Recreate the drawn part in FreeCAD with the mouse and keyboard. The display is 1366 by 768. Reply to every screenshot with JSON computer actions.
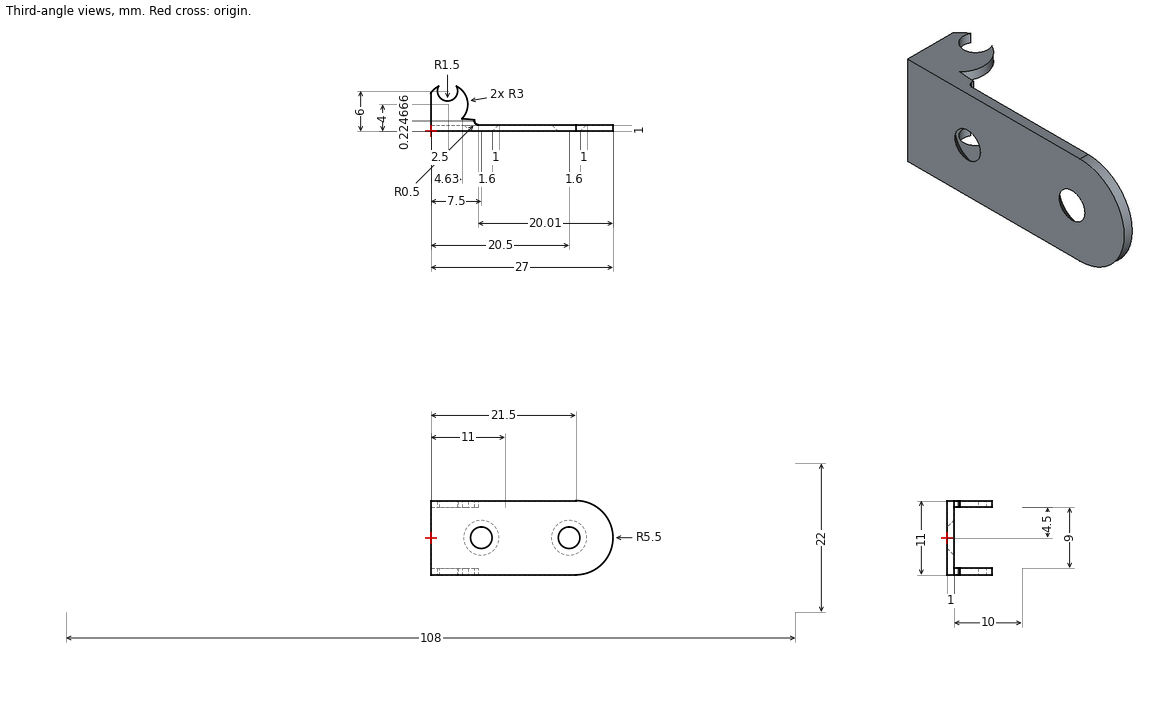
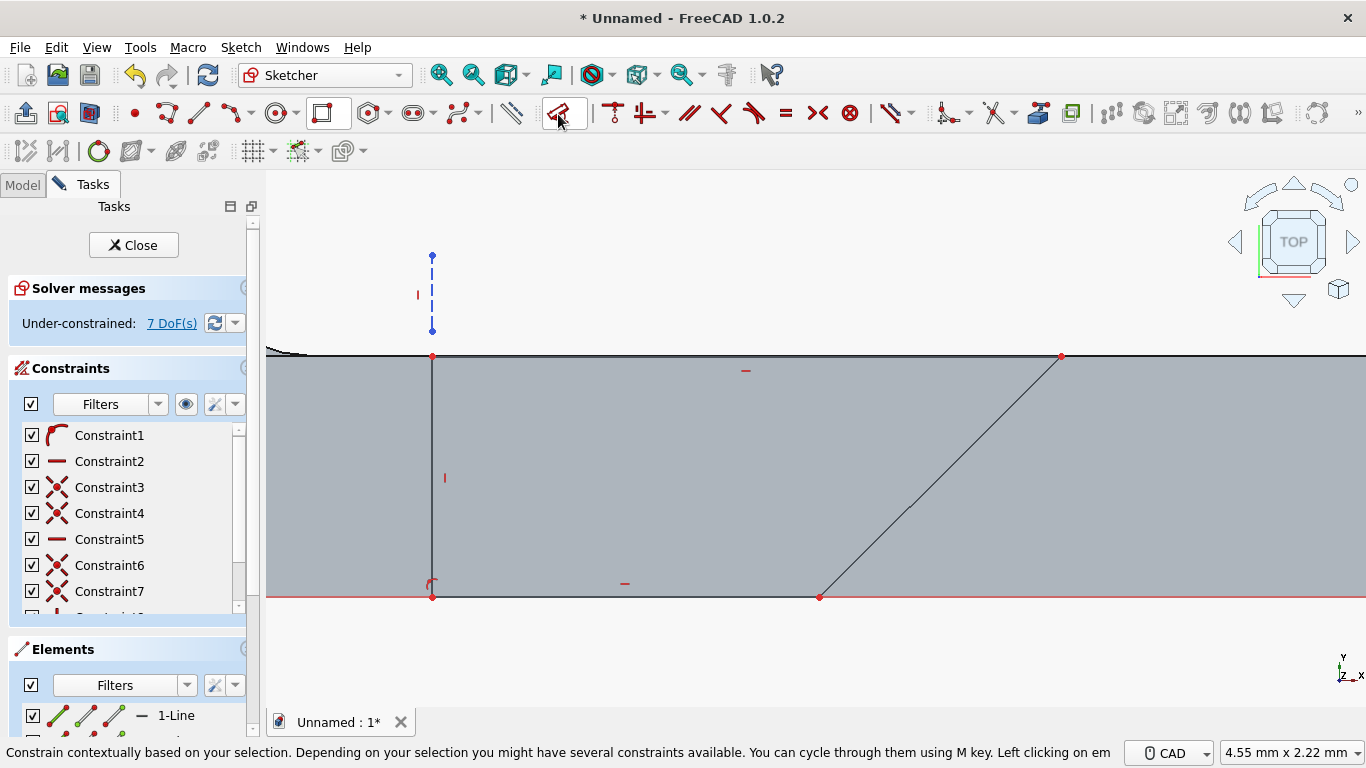
{"action": "left_click", "coordinate": [432, 429]}
{"action": "left_click", "coordinate": [398, 477]}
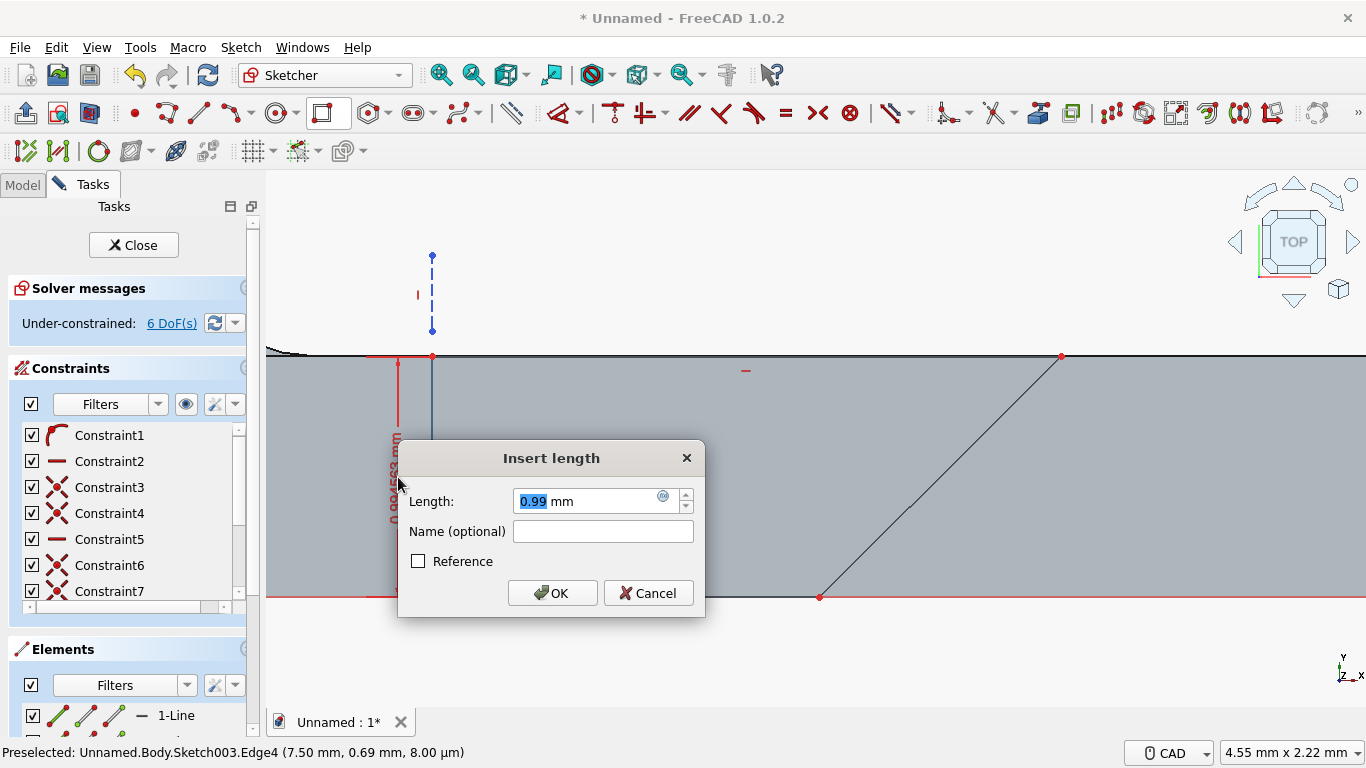
{"action": "type", "text": "1"}
{"action": "key", "text": "Return"}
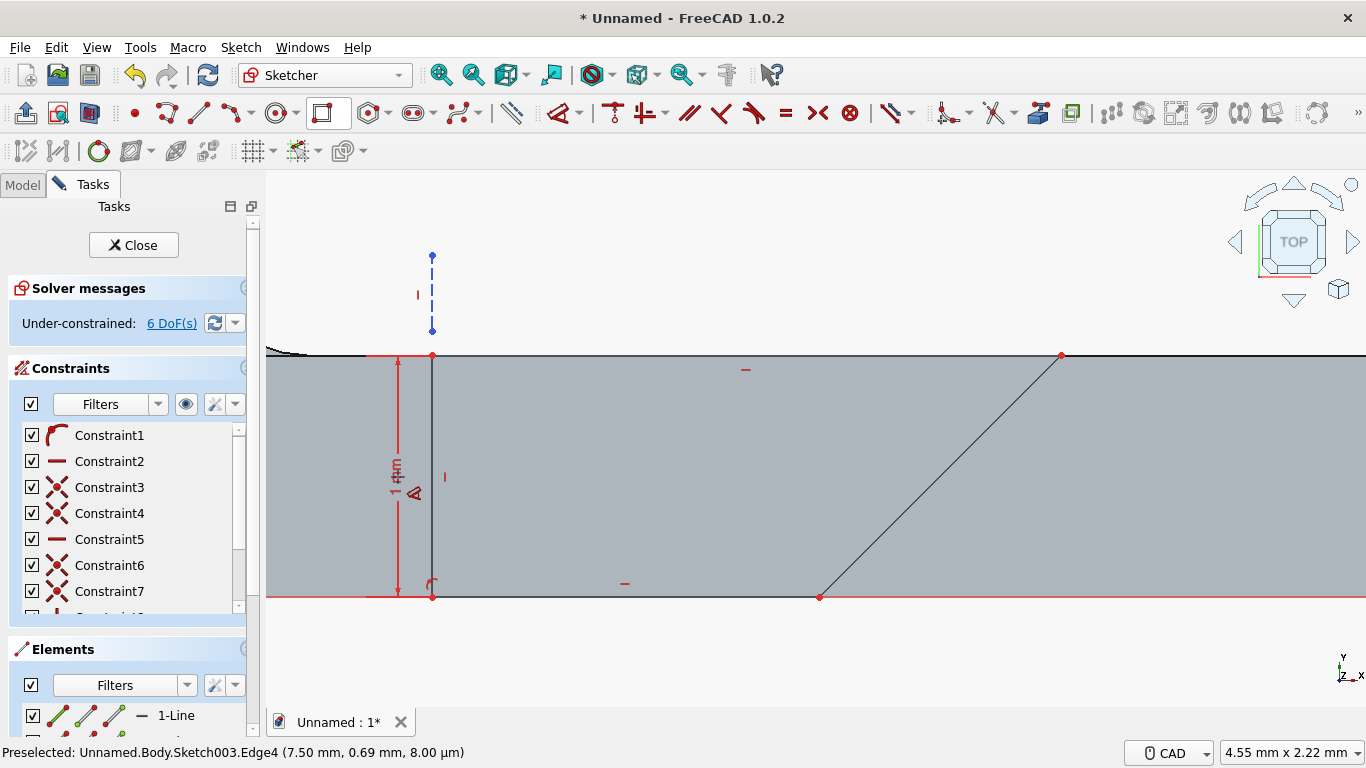
{"action": "left_click", "coordinate": [892, 525]}
{"action": "left_click", "coordinate": [940, 631]}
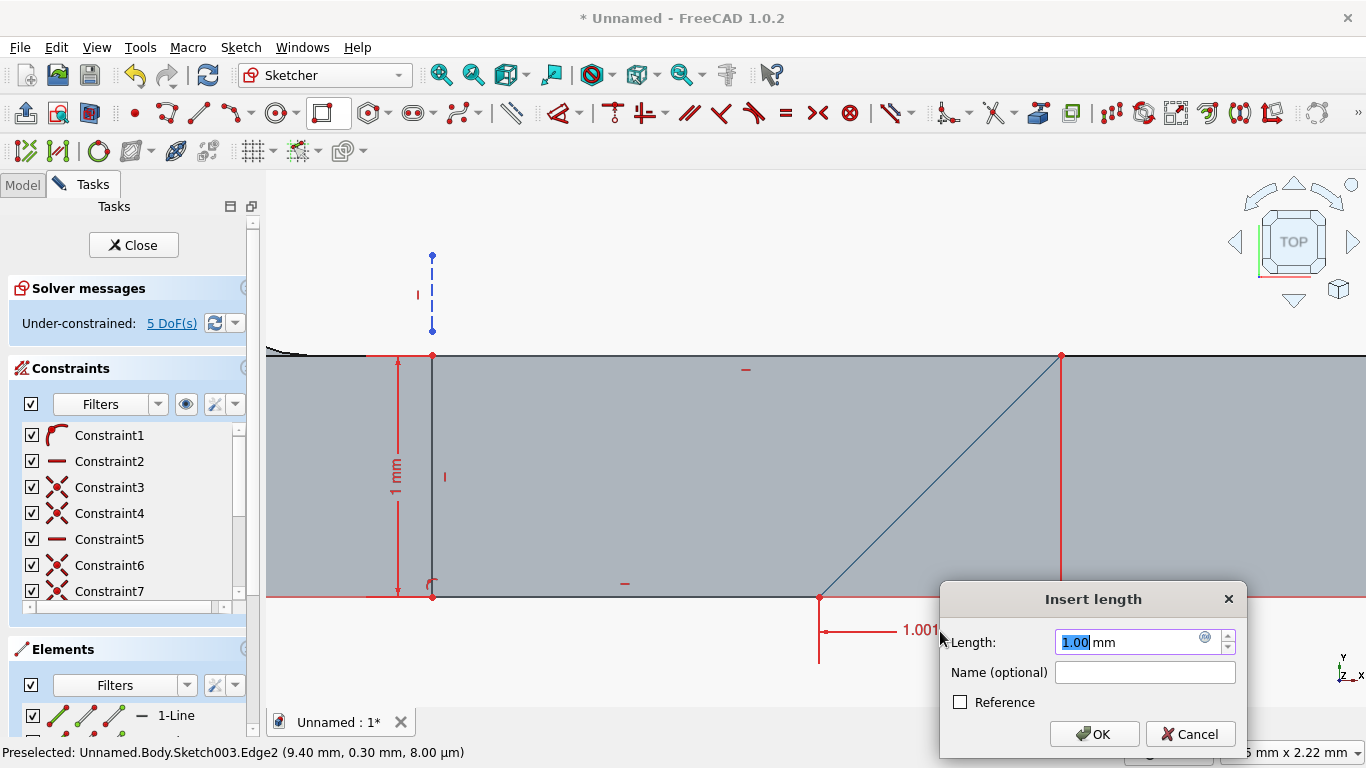
{"action": "type", "text": "1"}
{"action": "key", "text": "Return"}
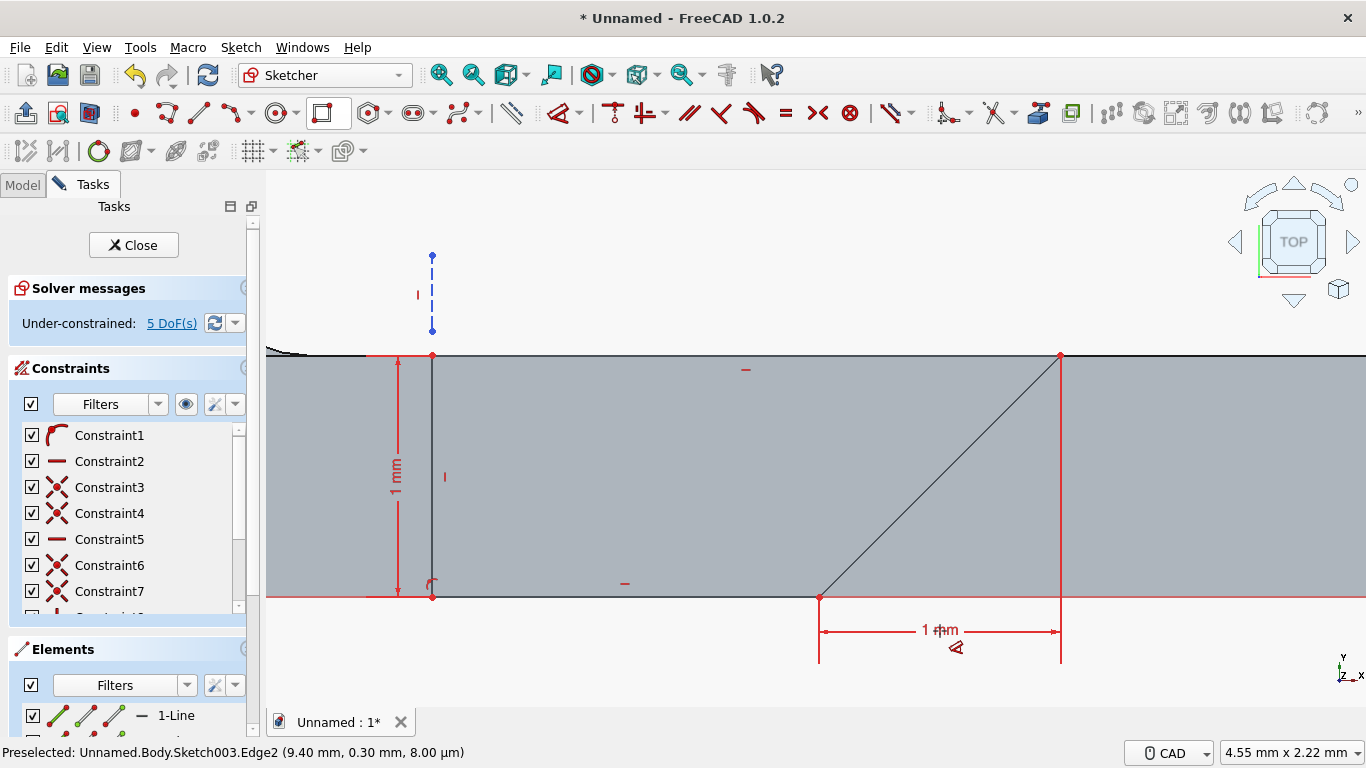
{"action": "left_click", "coordinate": [548, 597]}
{"action": "left_click", "coordinate": [625, 631]}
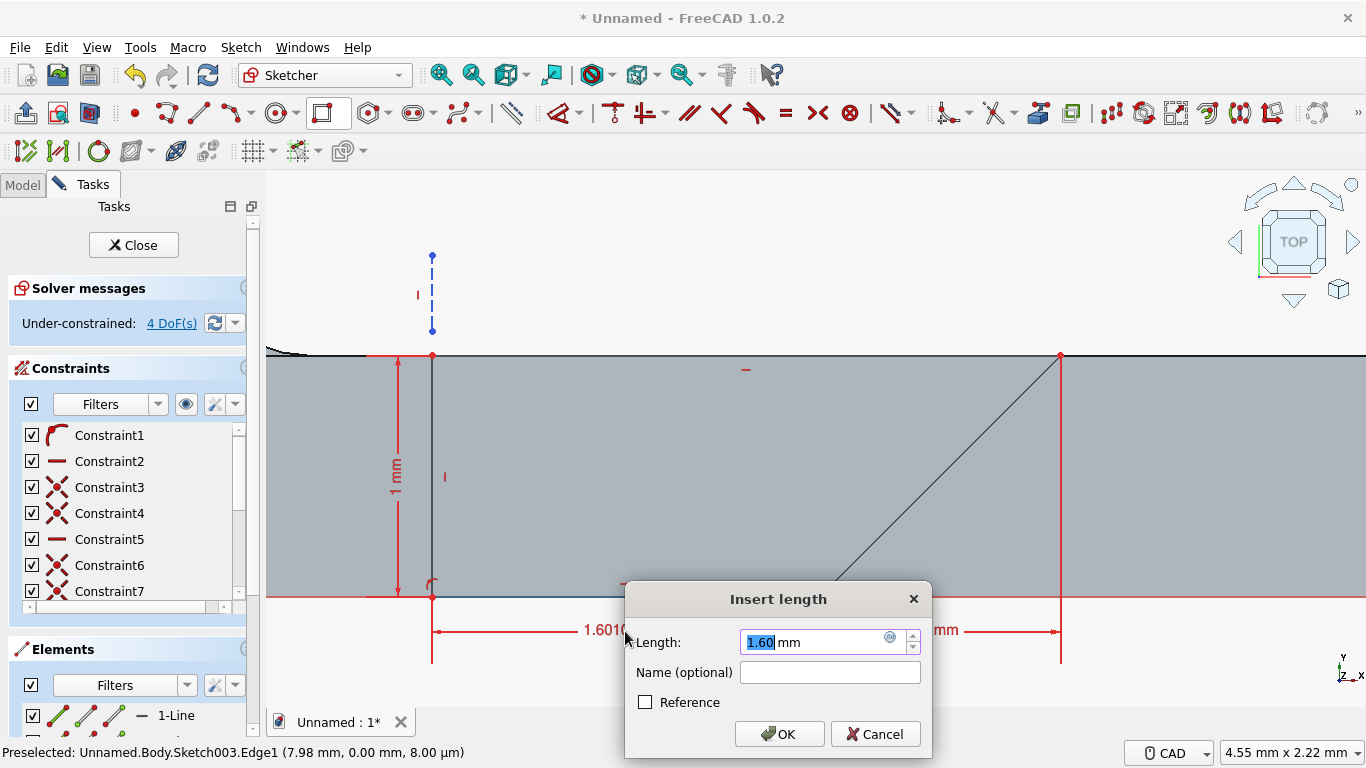
{"action": "type", "text": "1.6"}
{"action": "key", "text": "Return"}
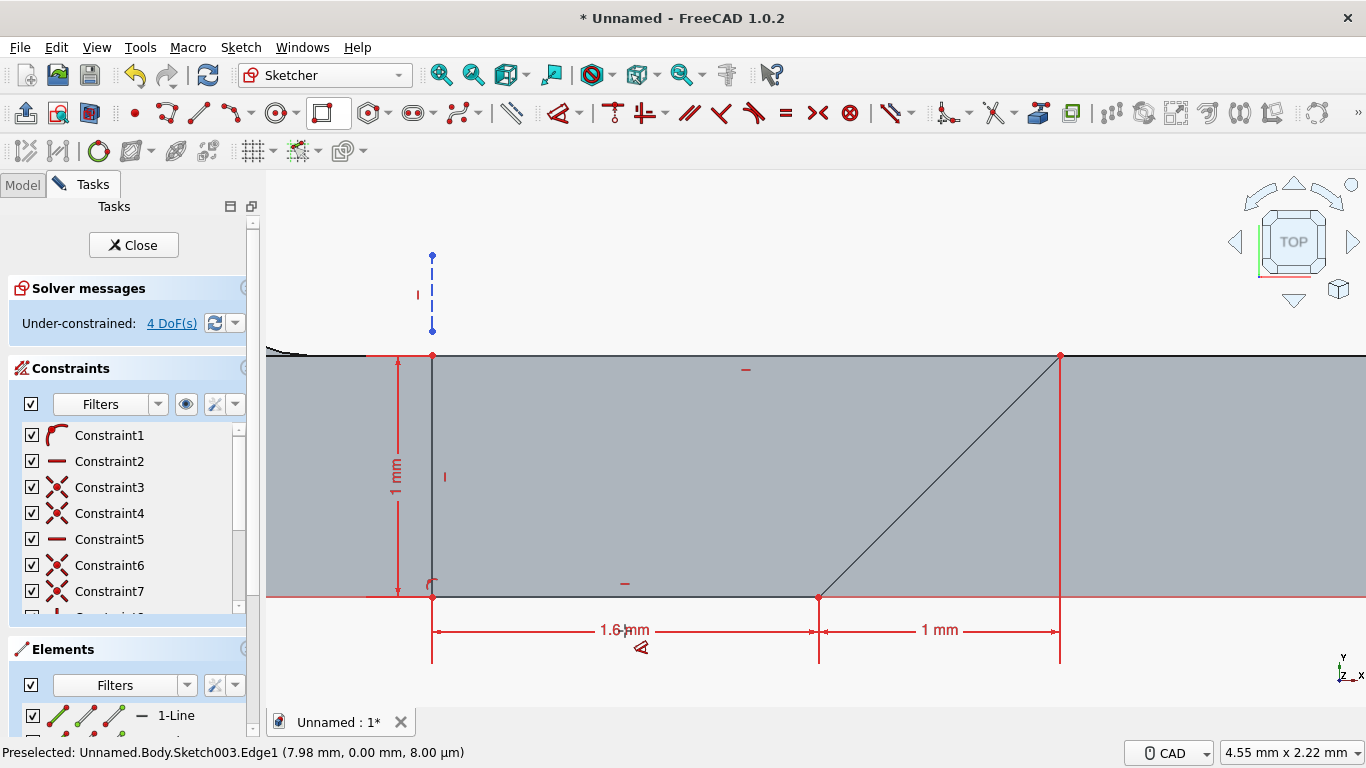
{"action": "left_click", "coordinate": [432, 597]}
{"action": "left_click", "coordinate": [363, 631]}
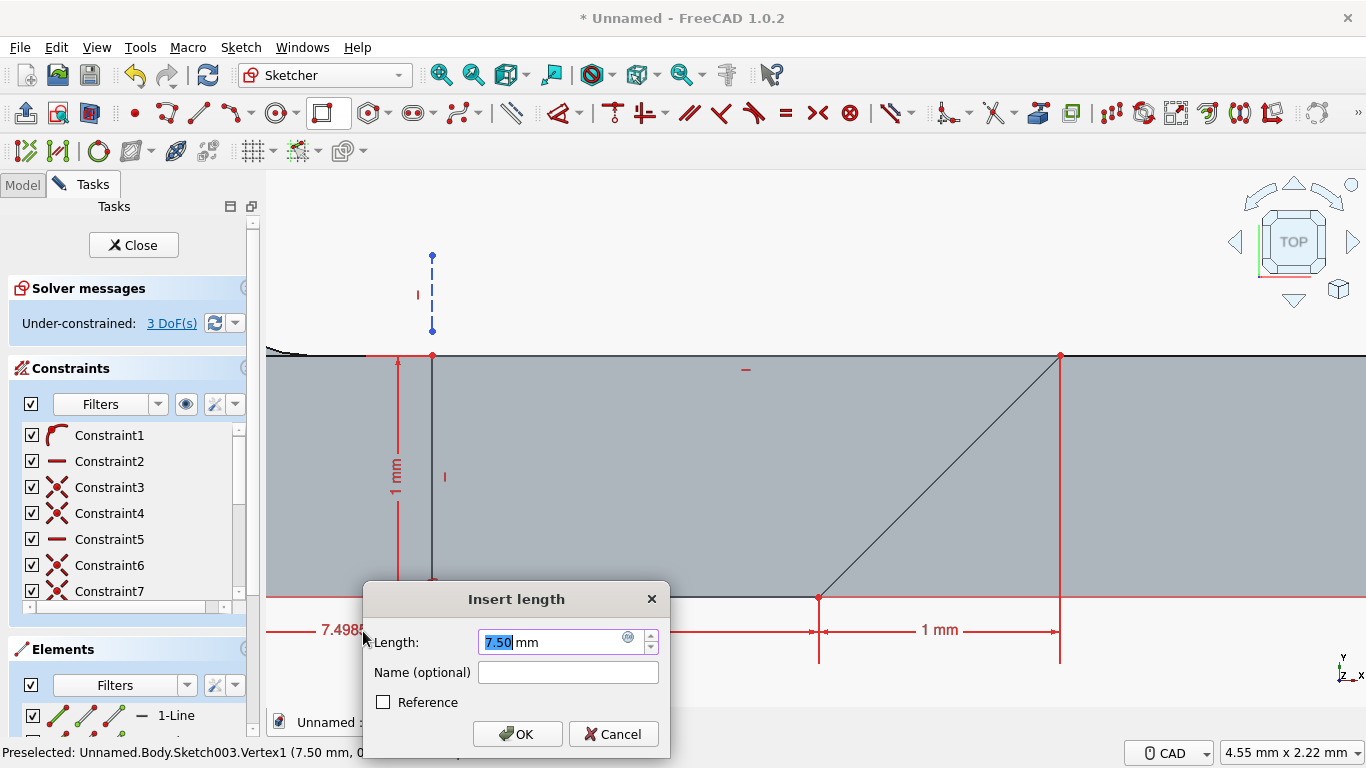
{"action": "type", "text": "7.5"}
{"action": "key", "text": "Return"}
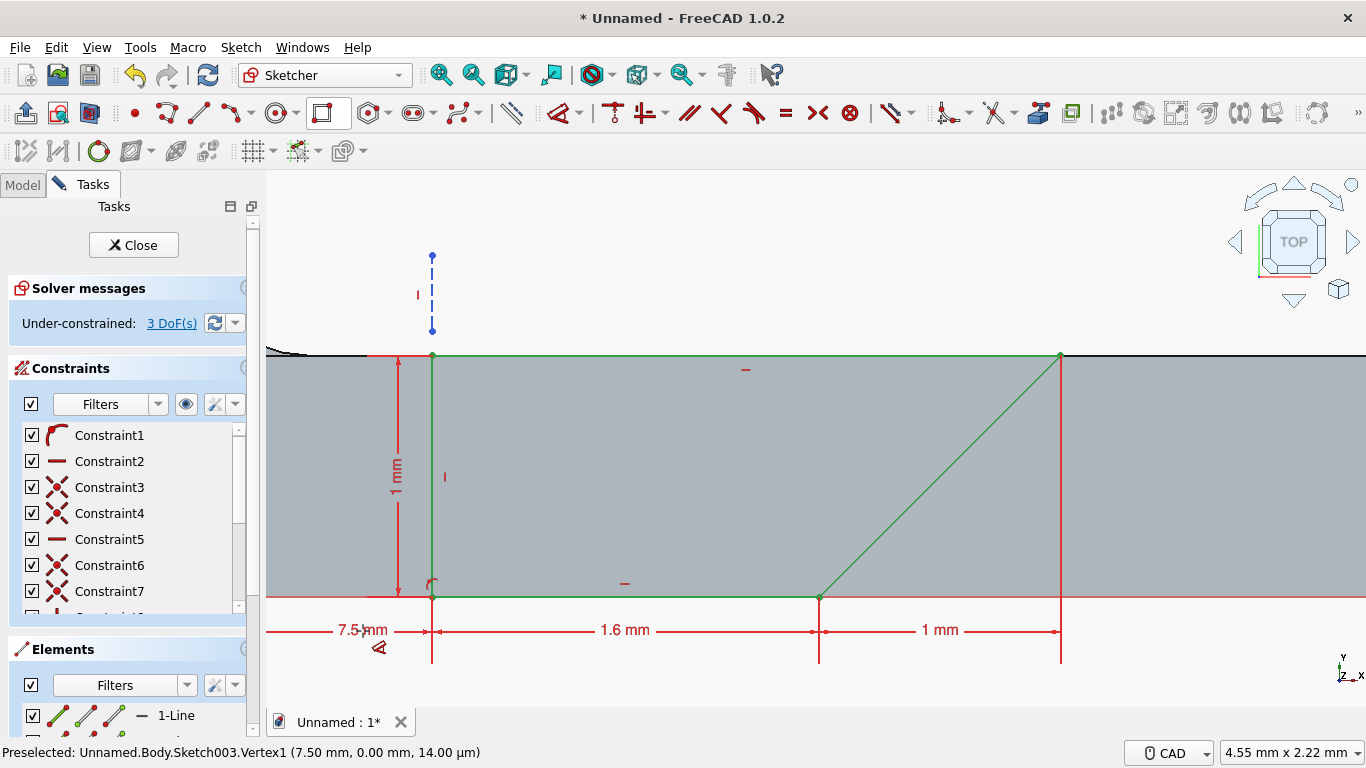
{"action": "left_click", "coordinate": [432, 332]}
{"action": "left_click", "coordinate": [363, 298]}